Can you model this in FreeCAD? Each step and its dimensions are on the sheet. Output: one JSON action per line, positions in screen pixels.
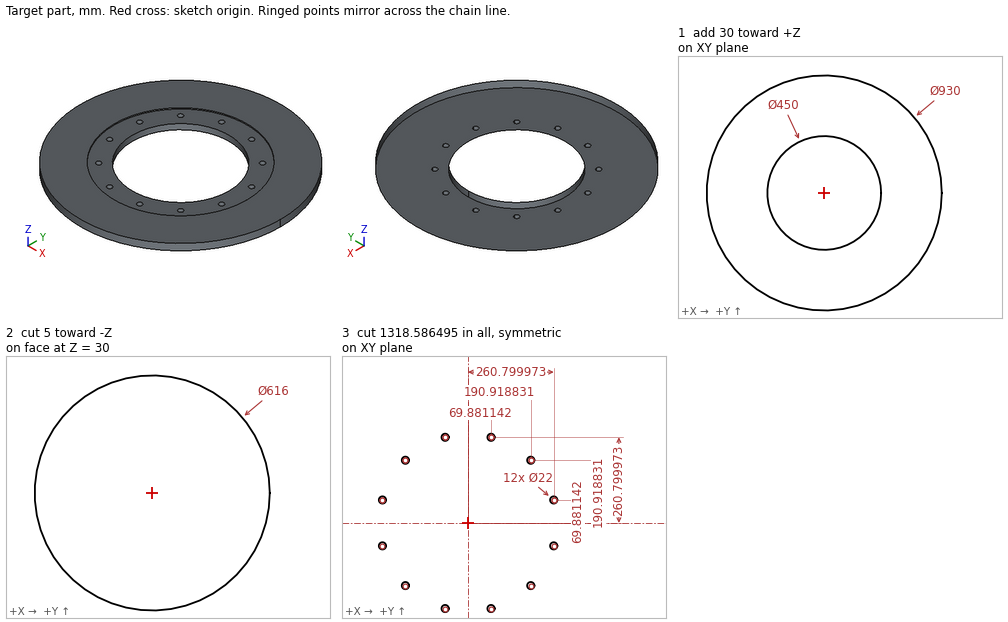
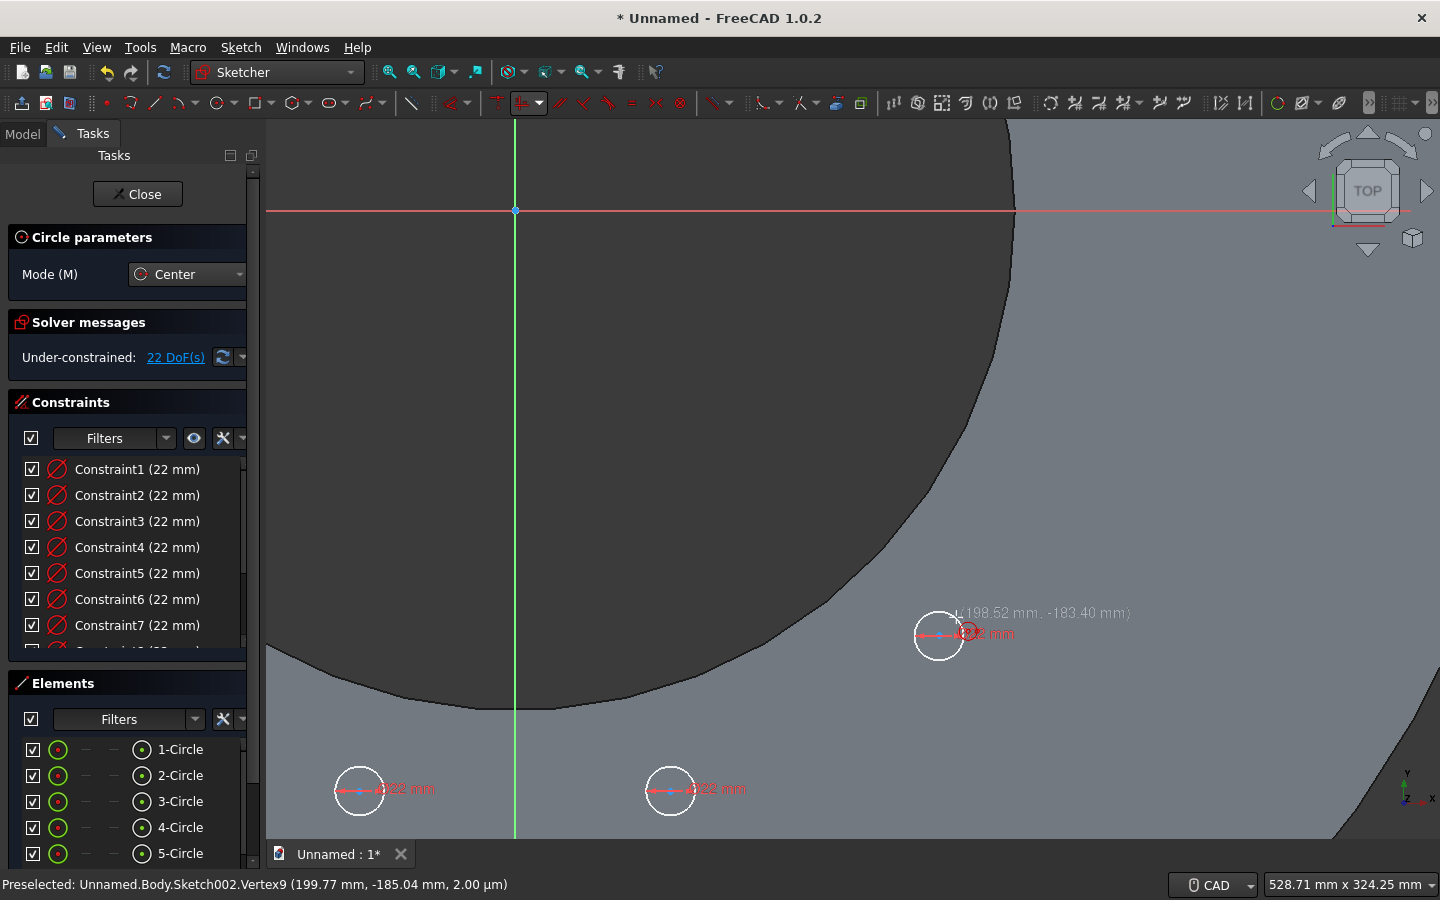
{"action": "left_click", "coordinate": [1094, 366]}
{"action": "mouse_move", "coordinate": [1112, 349]}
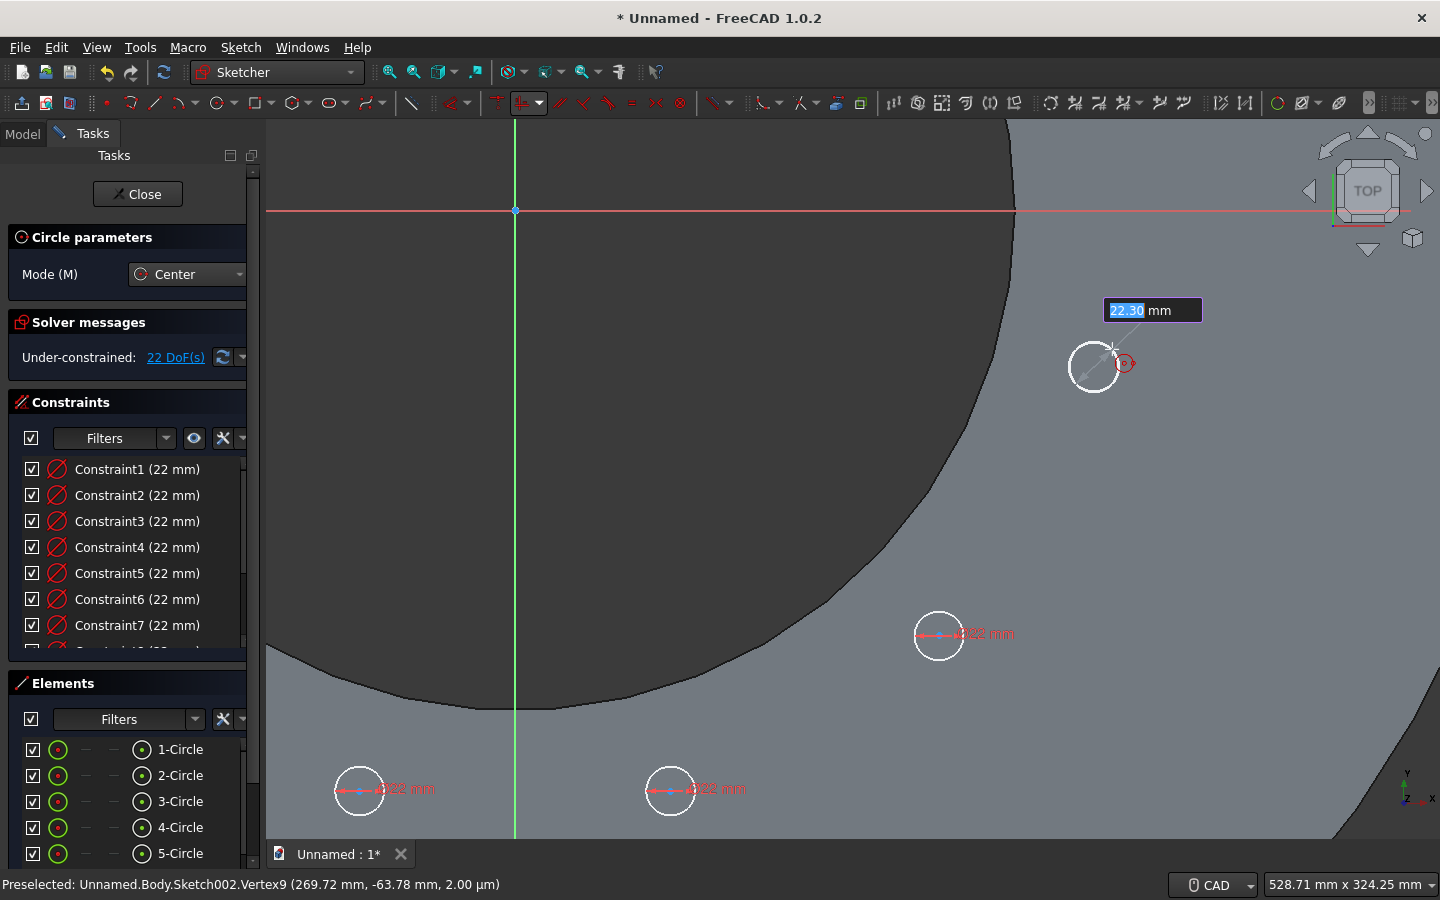
{"action": "type", "text": "22"}
{"action": "key", "text": "Return"}
{"action": "key", "text": "Escape"}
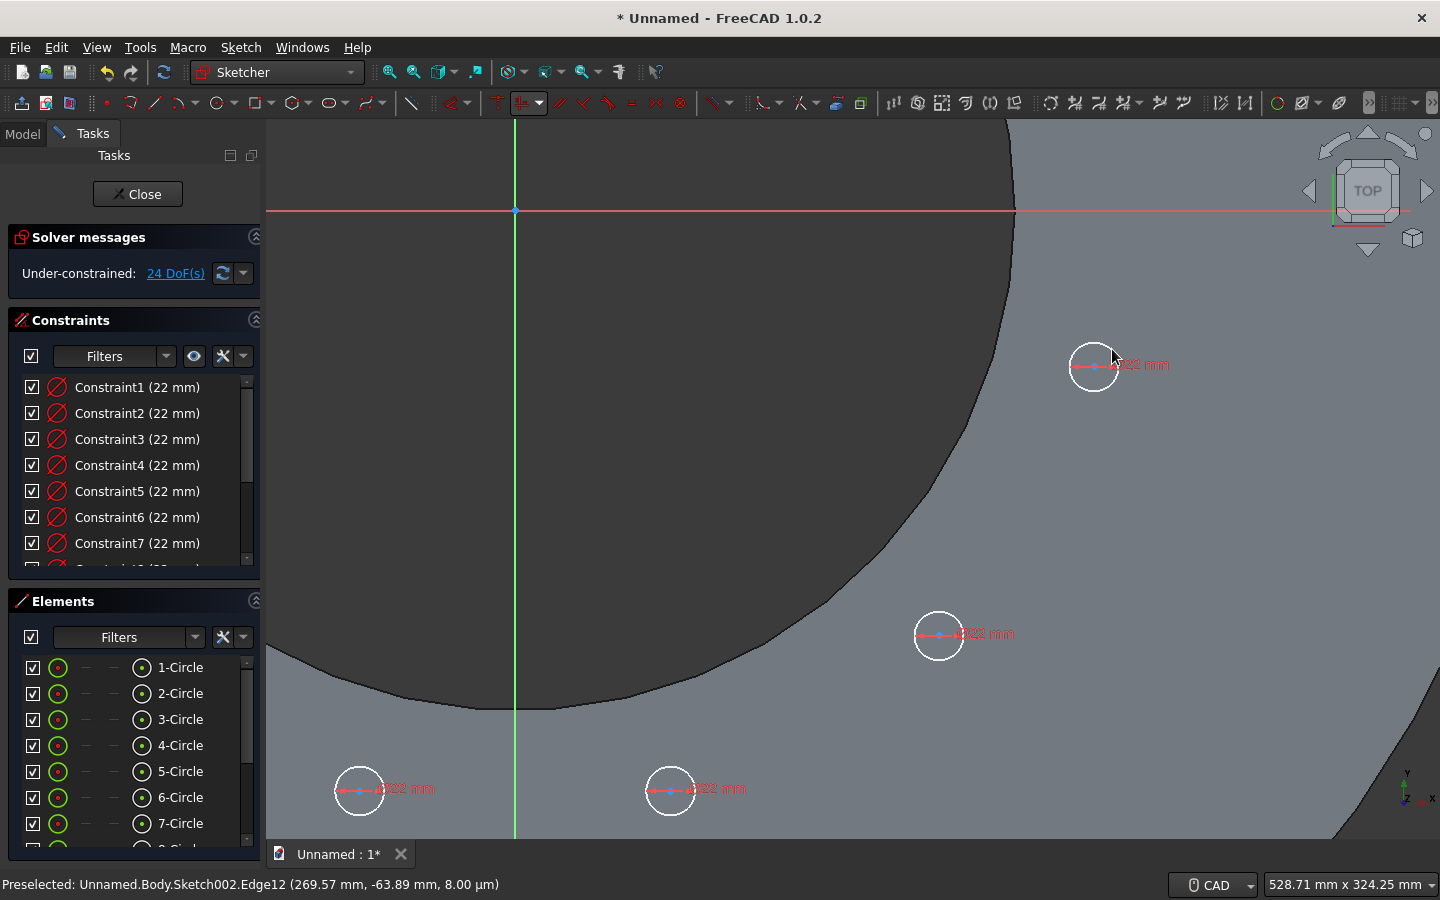
{"action": "scroll", "coordinate": [941, 635], "scroll_direction": "down", "scroll_amount": 5}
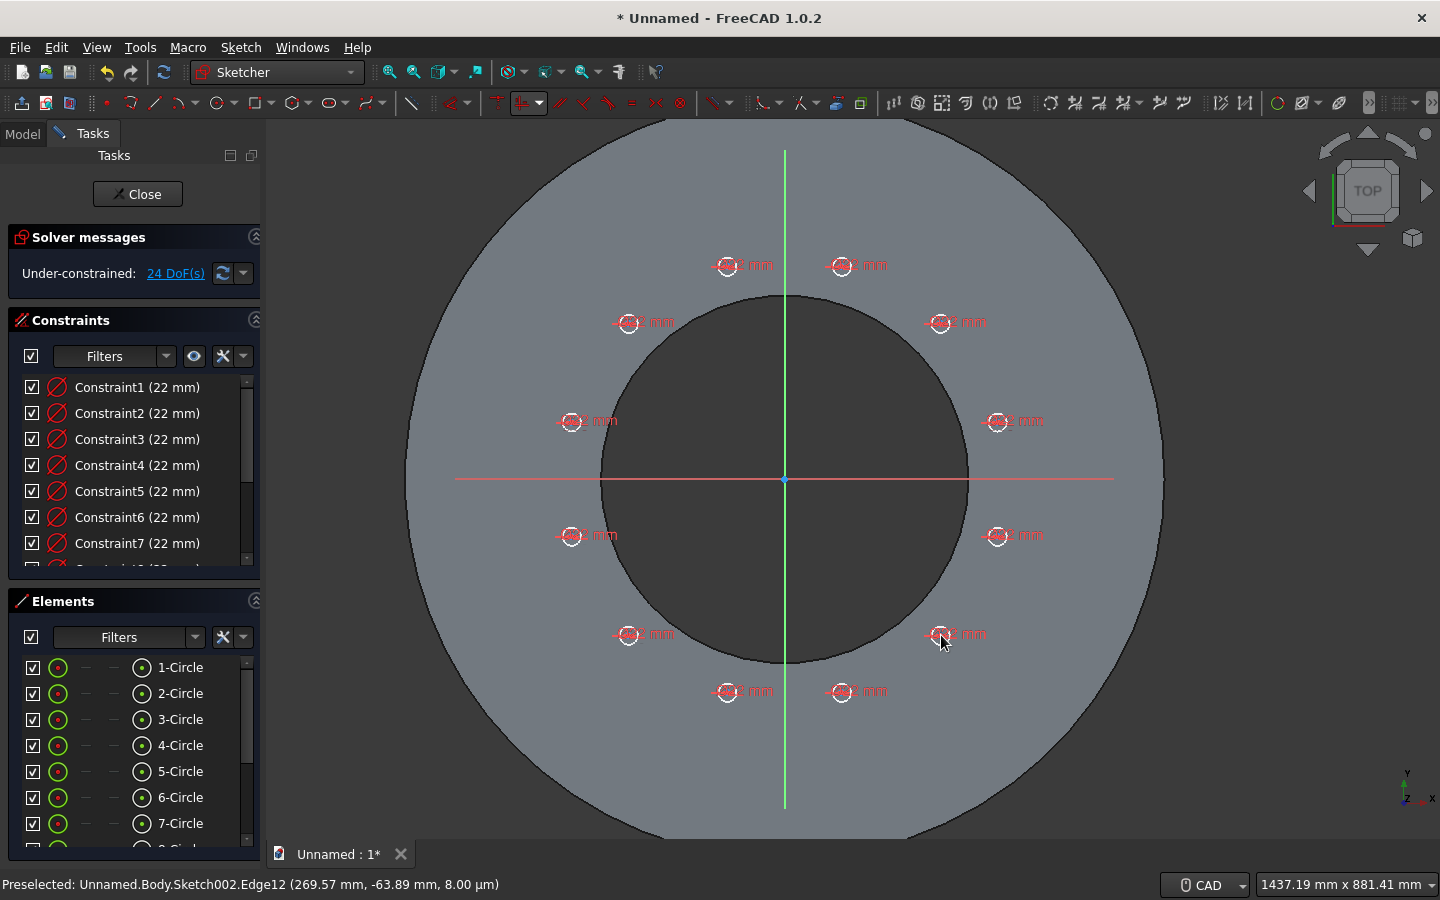
{"action": "left_click", "coordinate": [842, 267]}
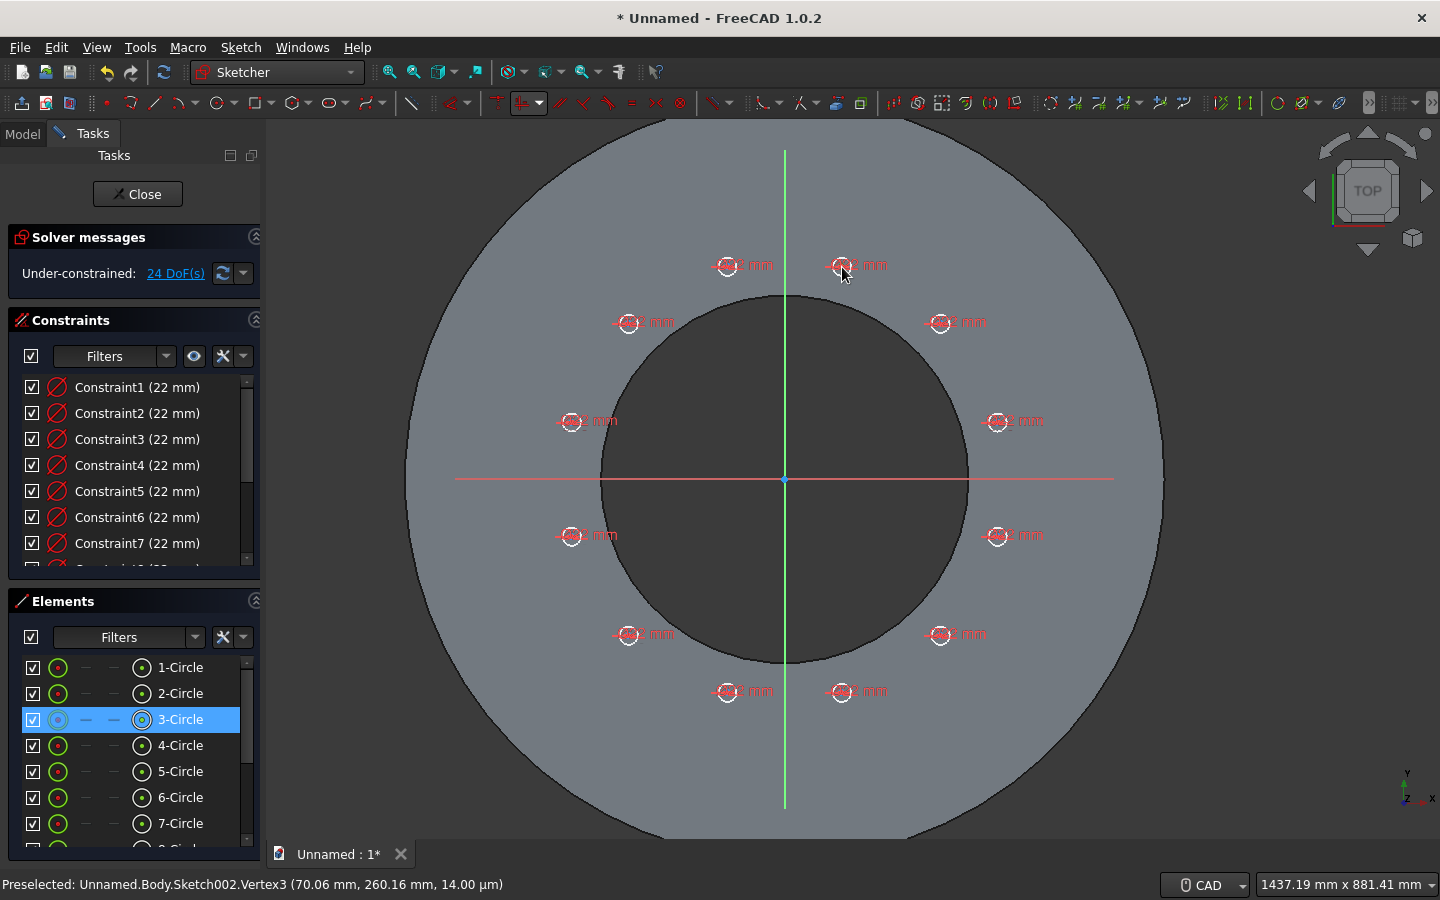
{"action": "left_click", "coordinate": [728, 267]}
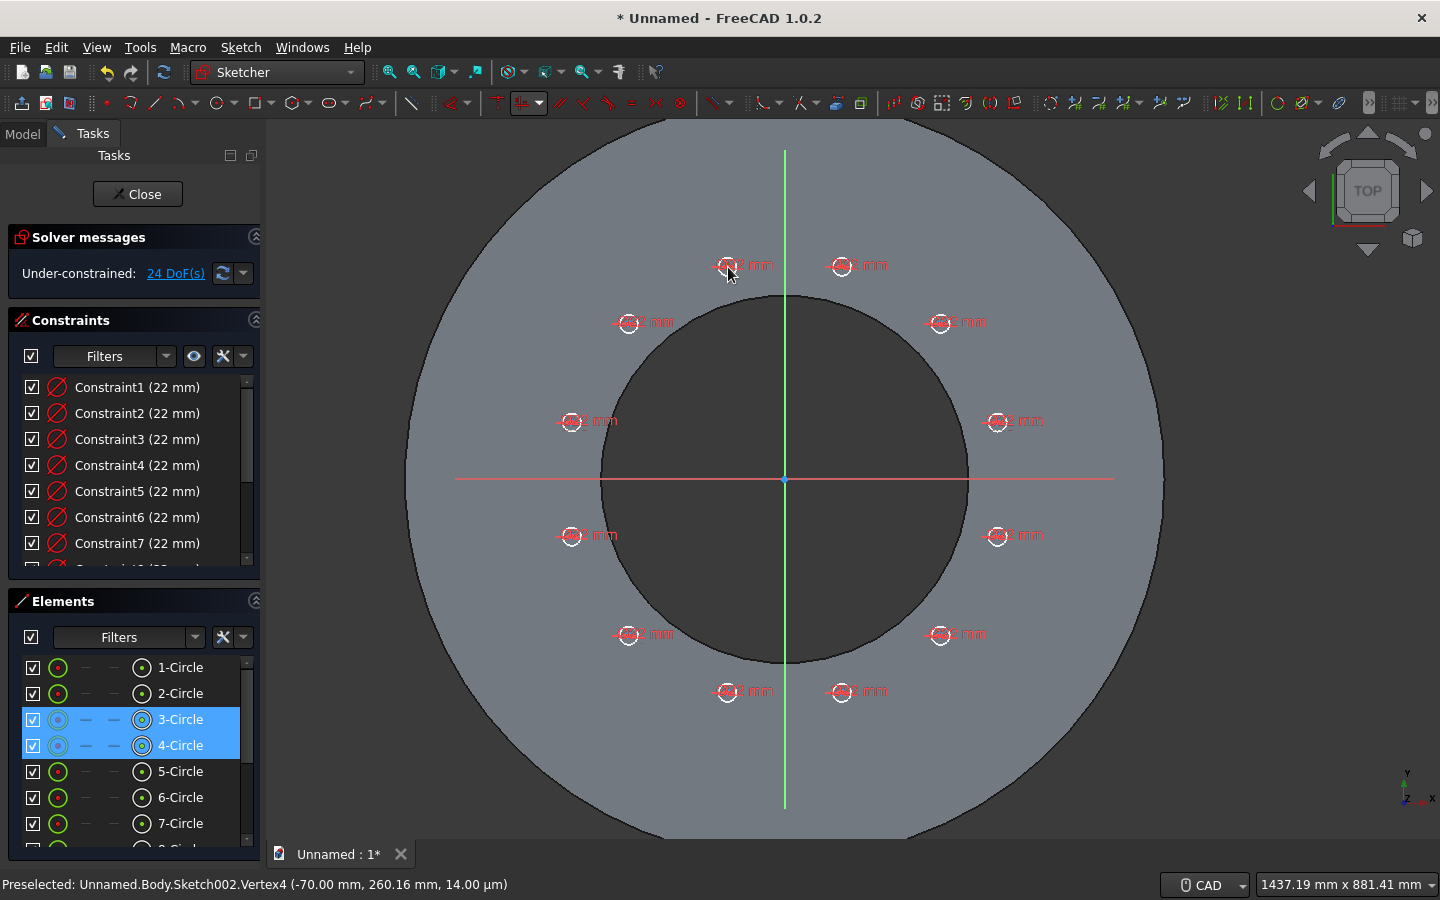
{"action": "left_click", "coordinate": [785, 764]}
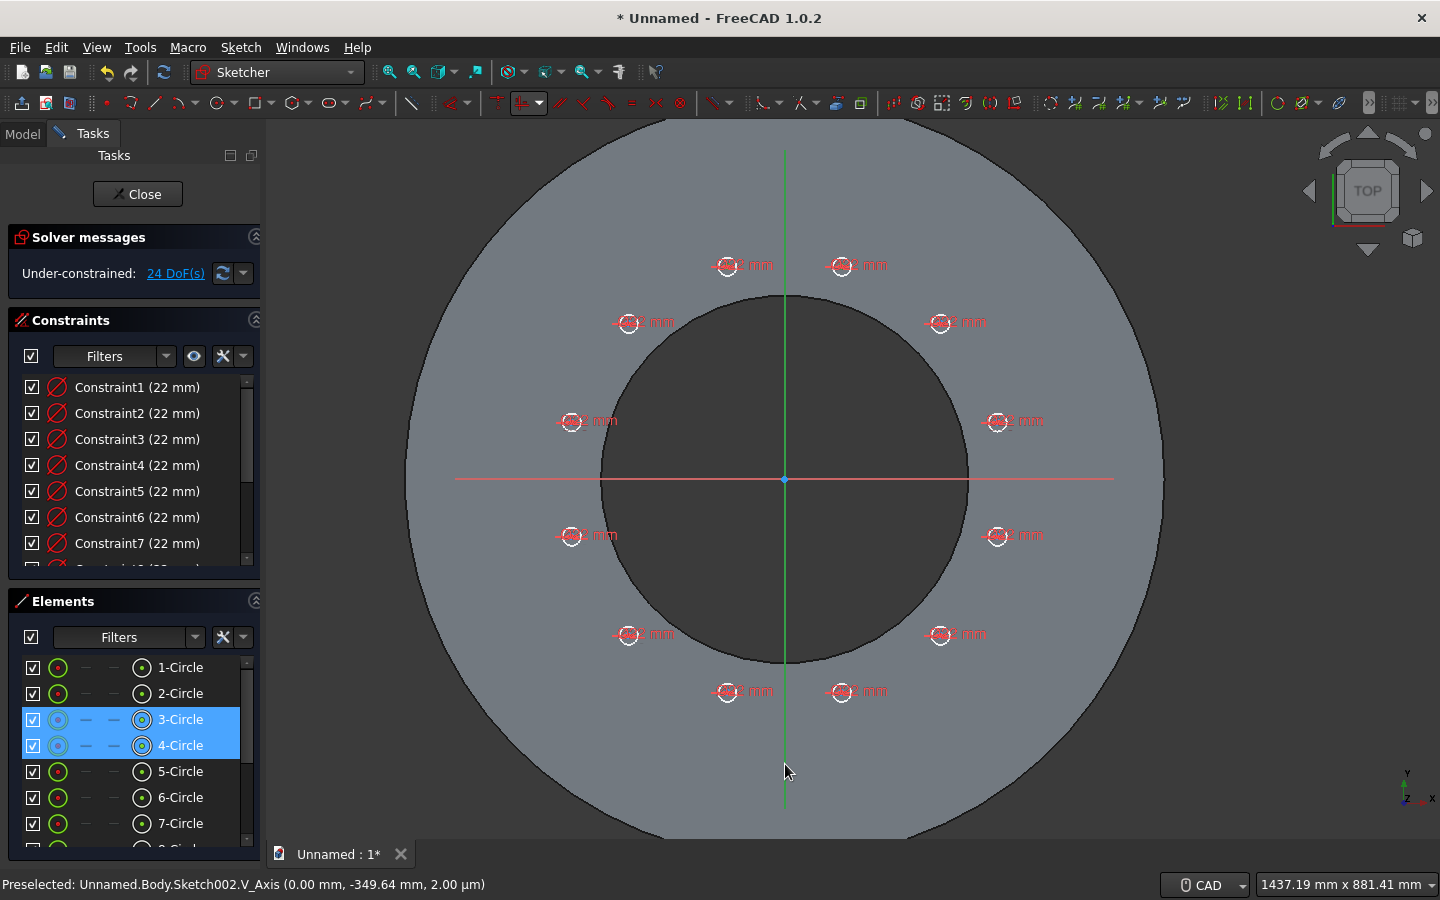
{"action": "left_click", "coordinate": [656, 104]}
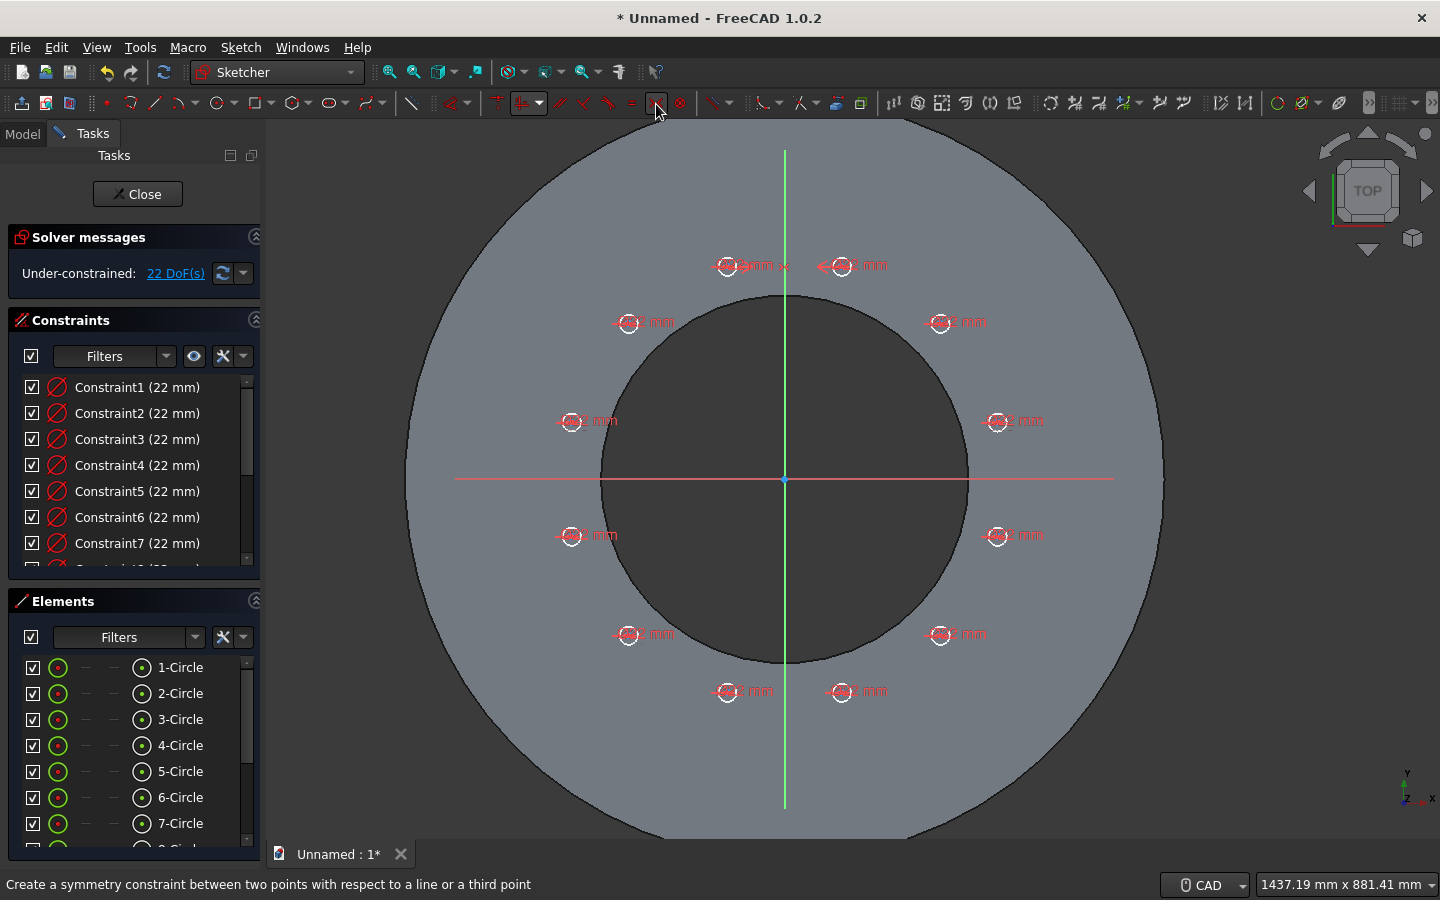
{"action": "left_click", "coordinate": [941, 324]}